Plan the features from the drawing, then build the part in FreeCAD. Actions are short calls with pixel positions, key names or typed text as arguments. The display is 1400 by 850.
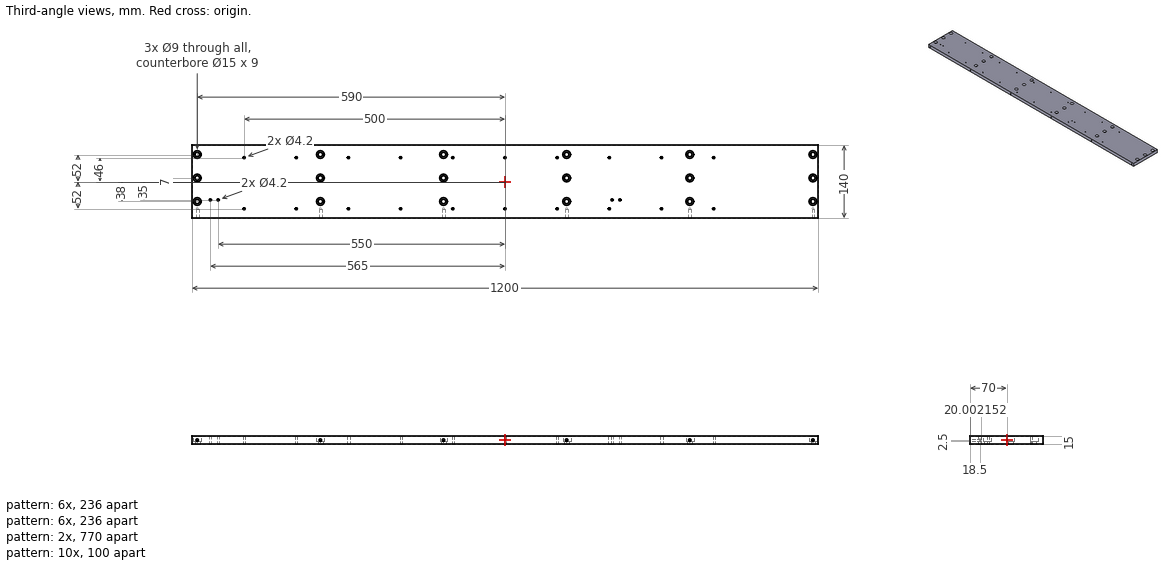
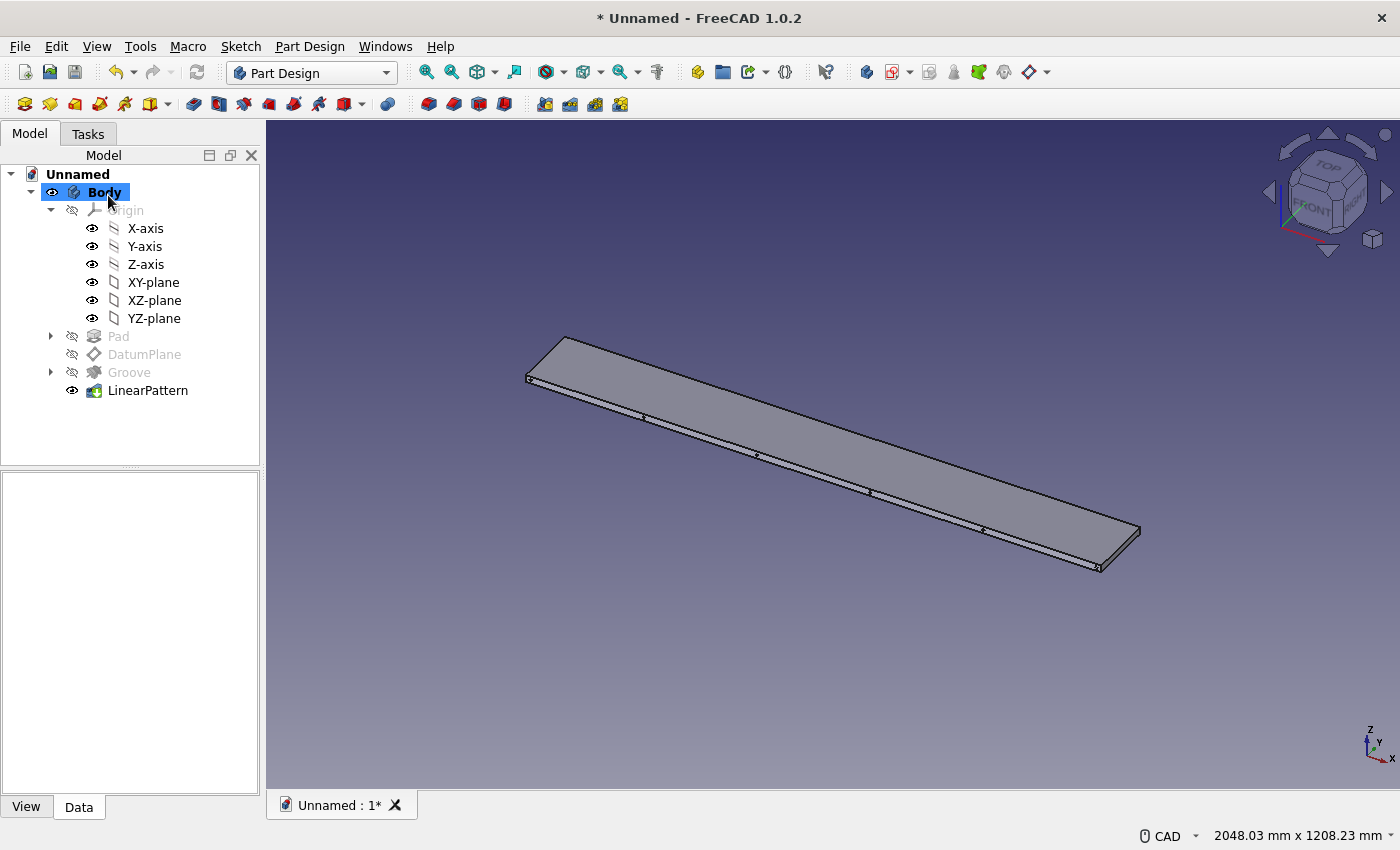
click(1080, 532)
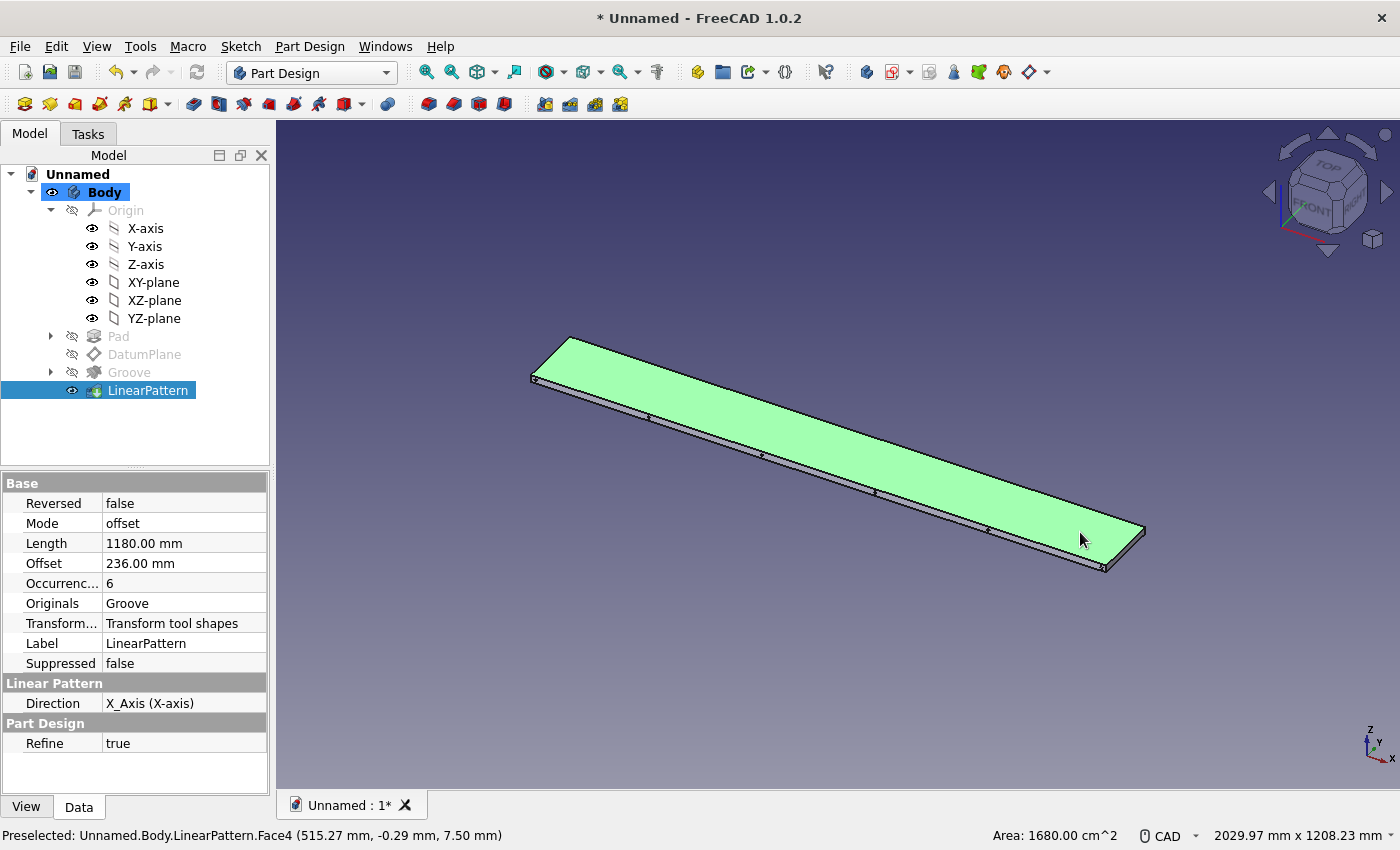
click(892, 72)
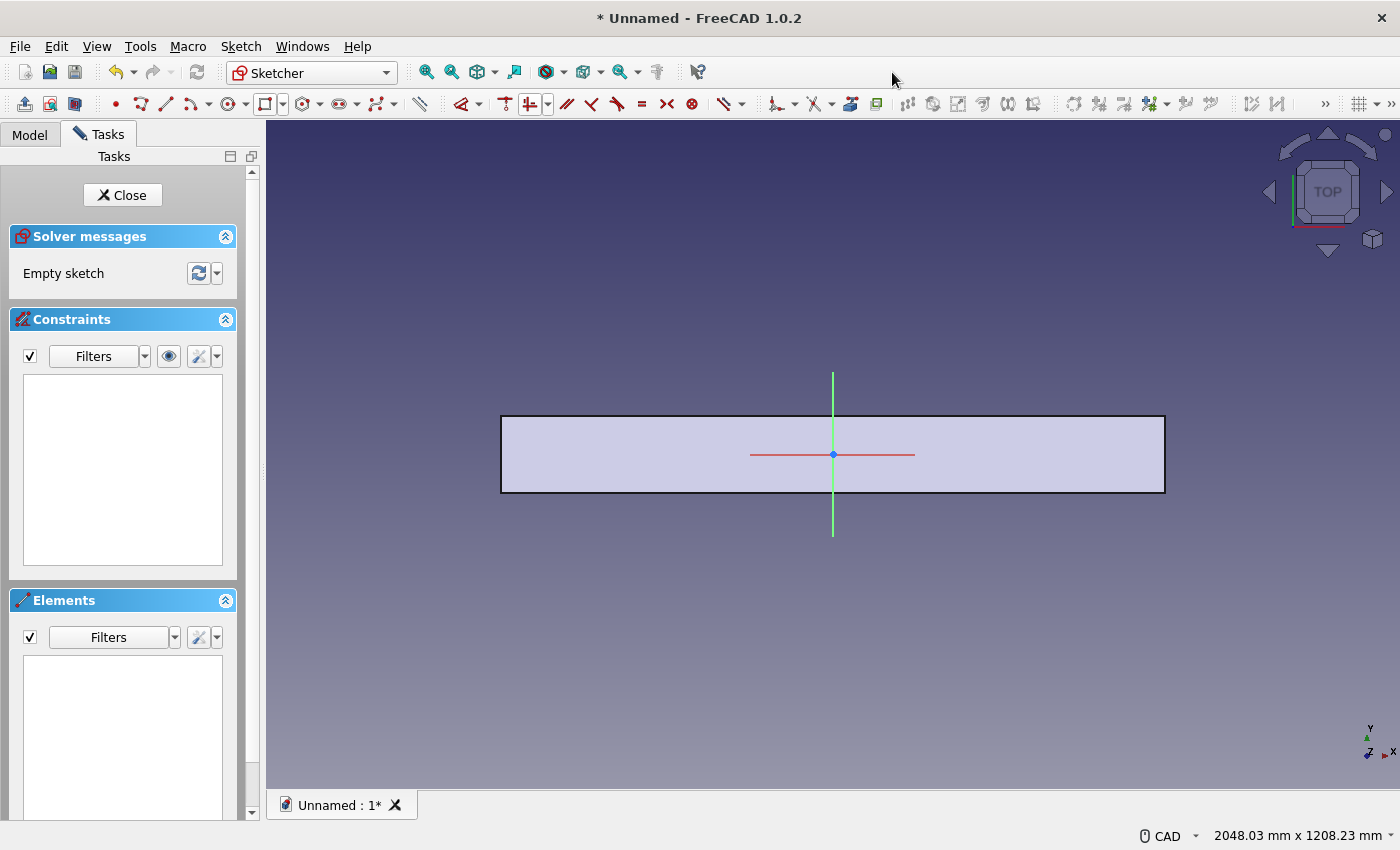
scroll(466, 450, up, 10)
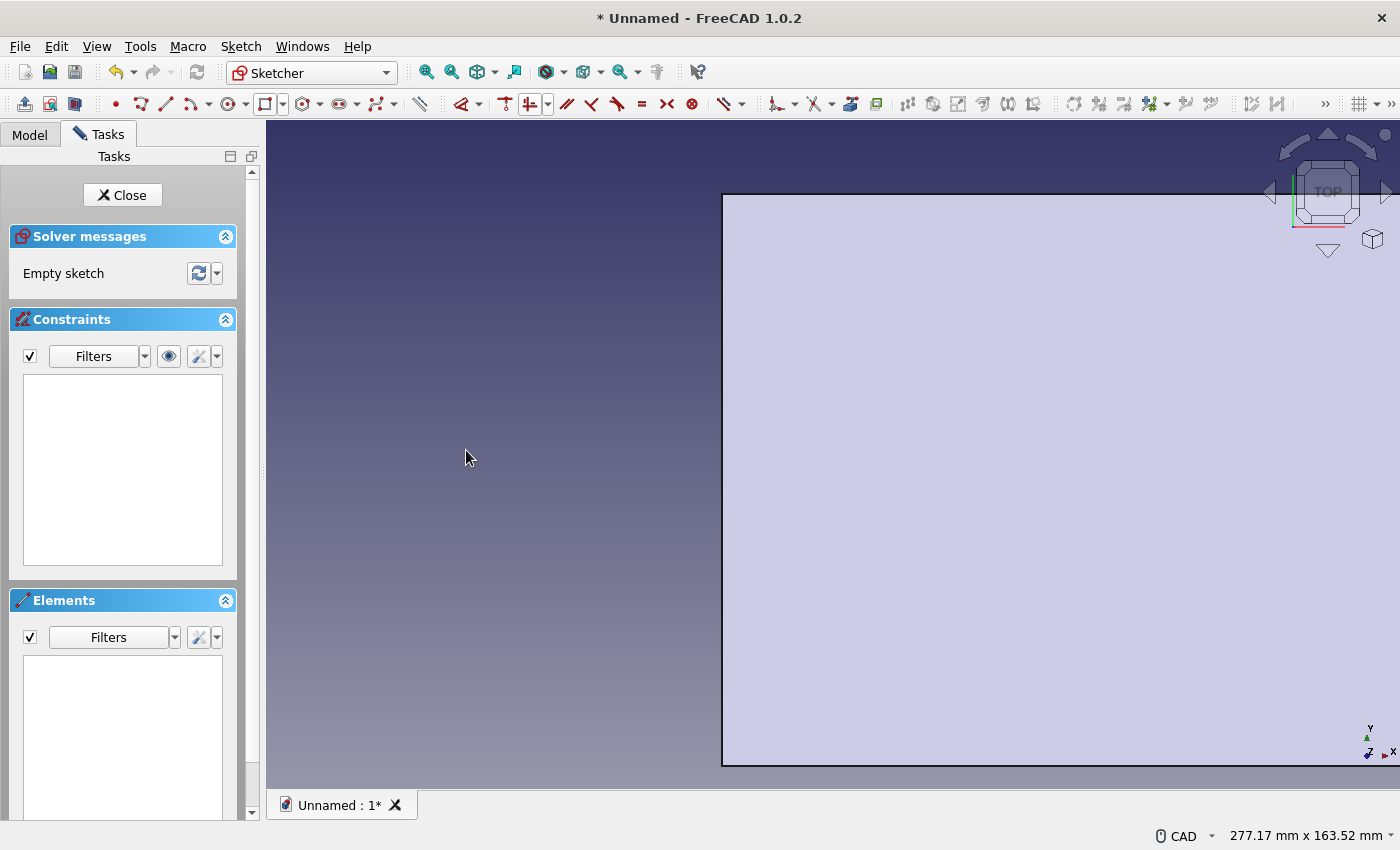
key(g)
key(c)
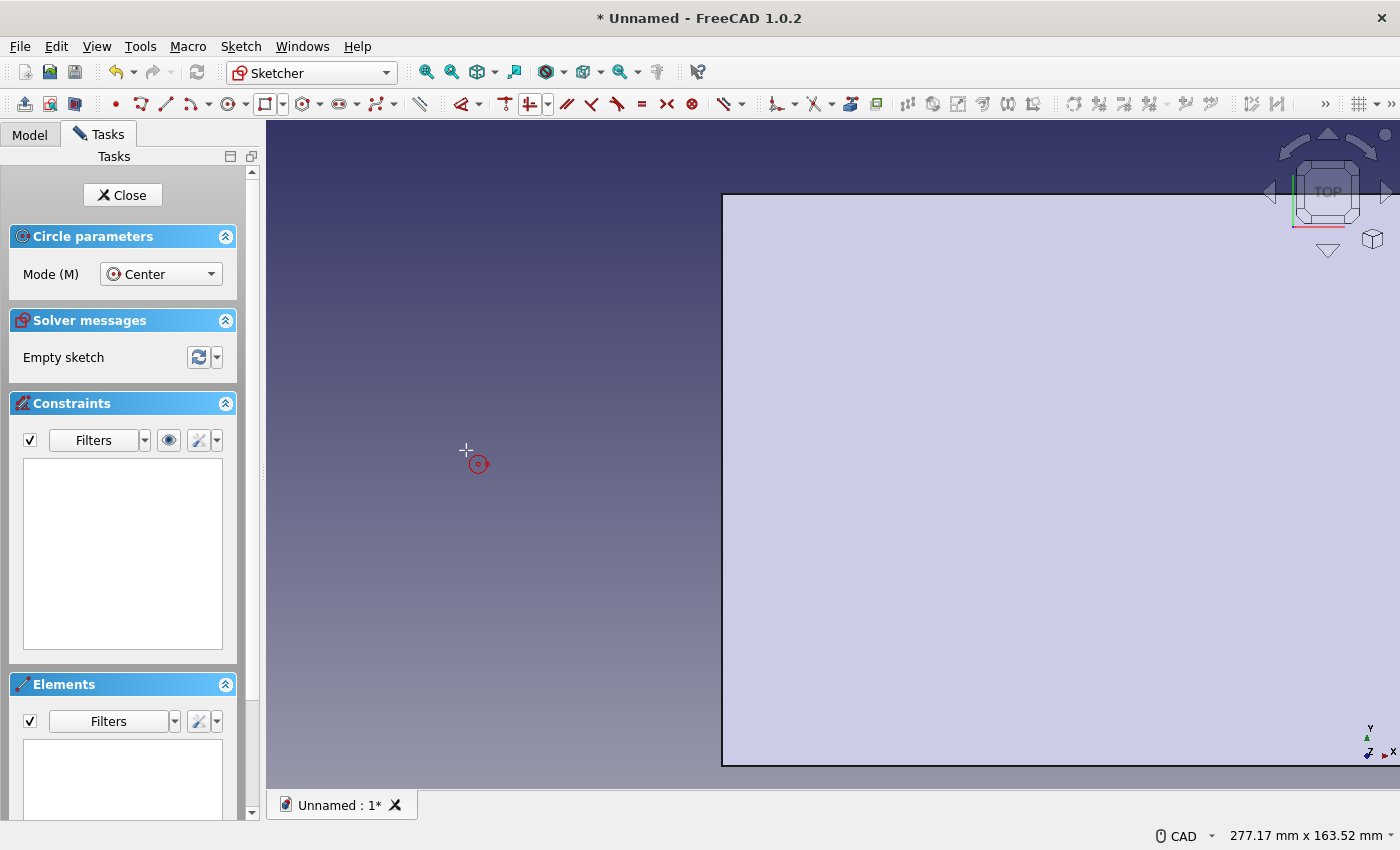
scroll(763, 267, up, 2)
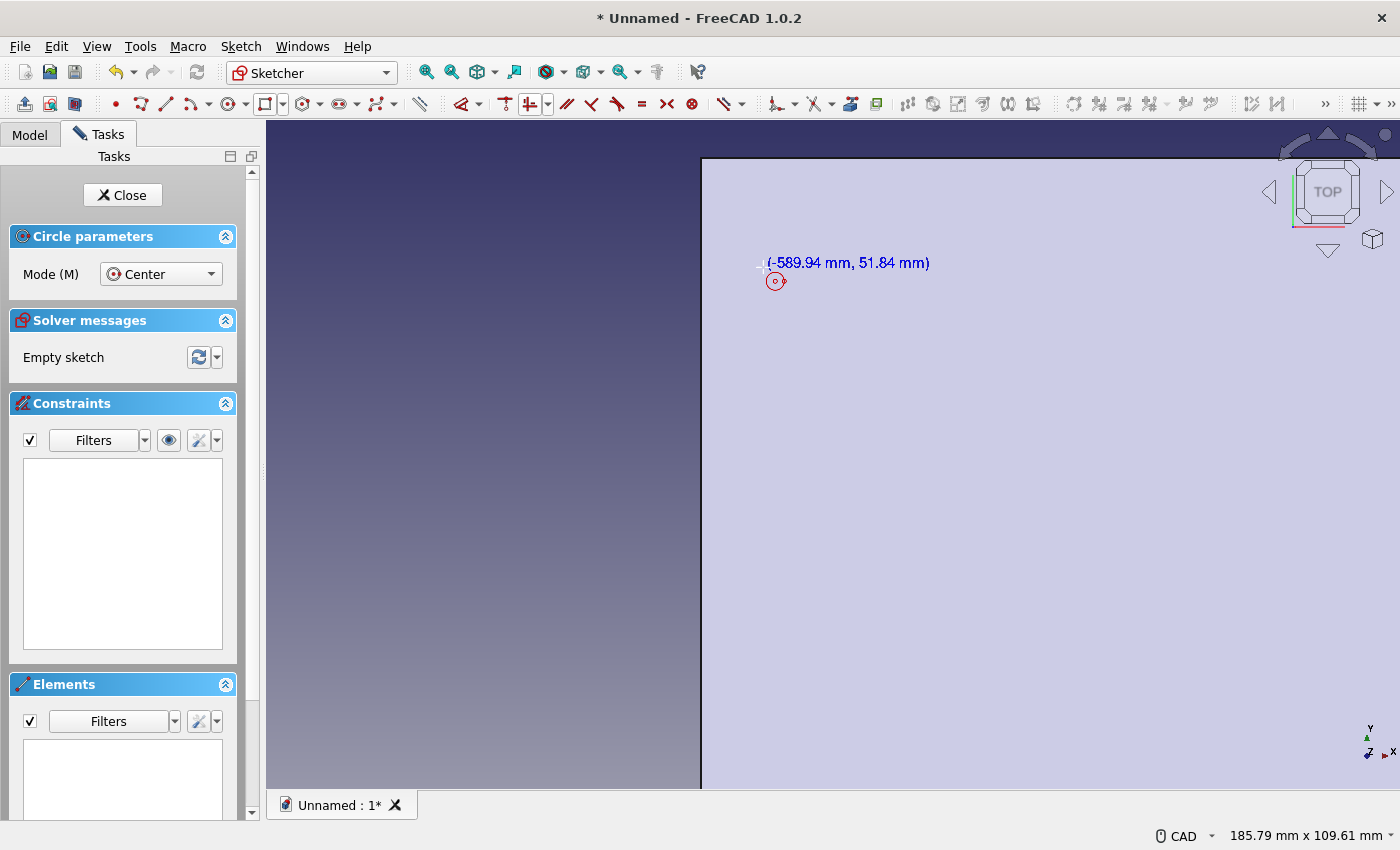
click(762, 267)
move(782, 248)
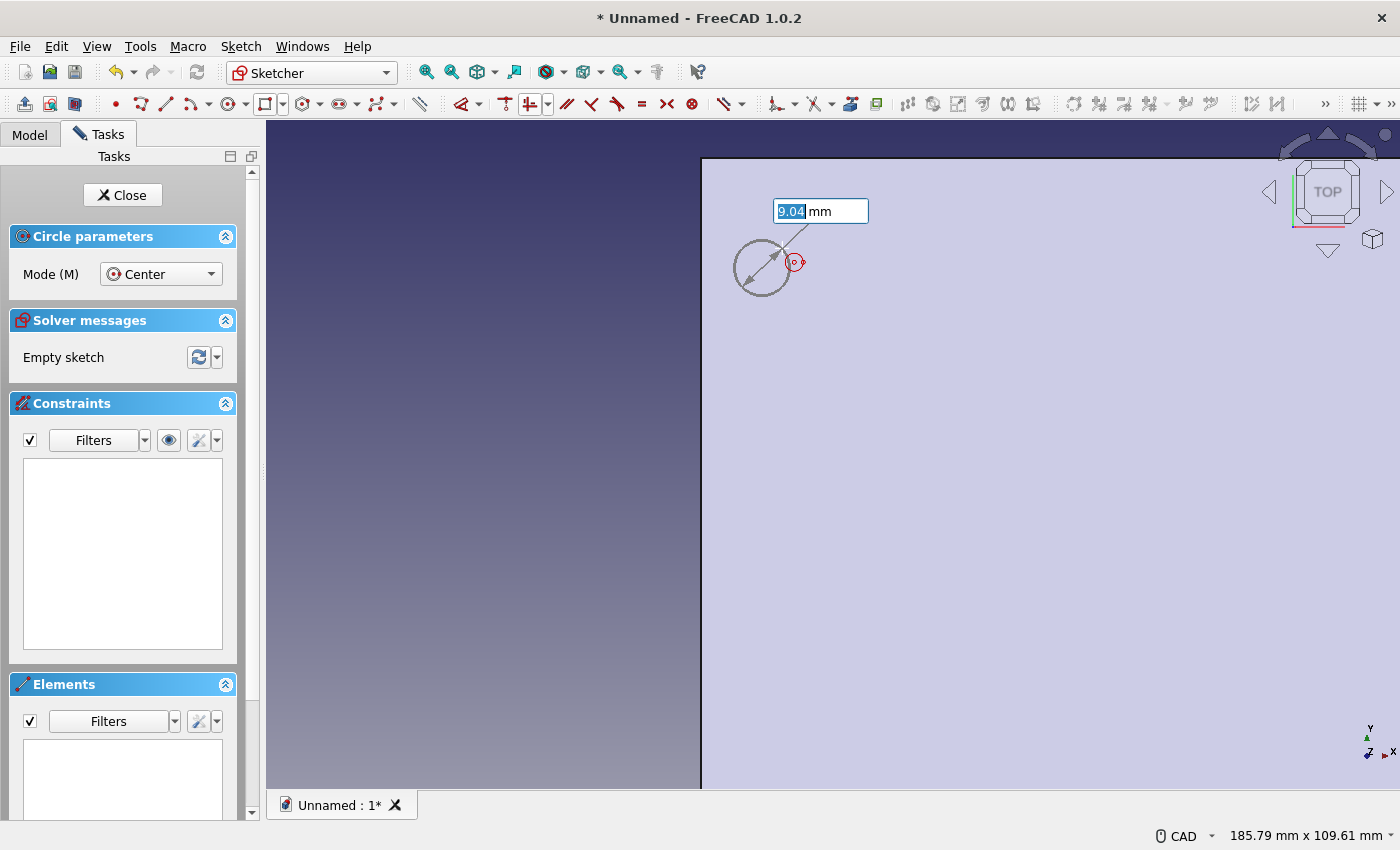
text(9)
key(Return)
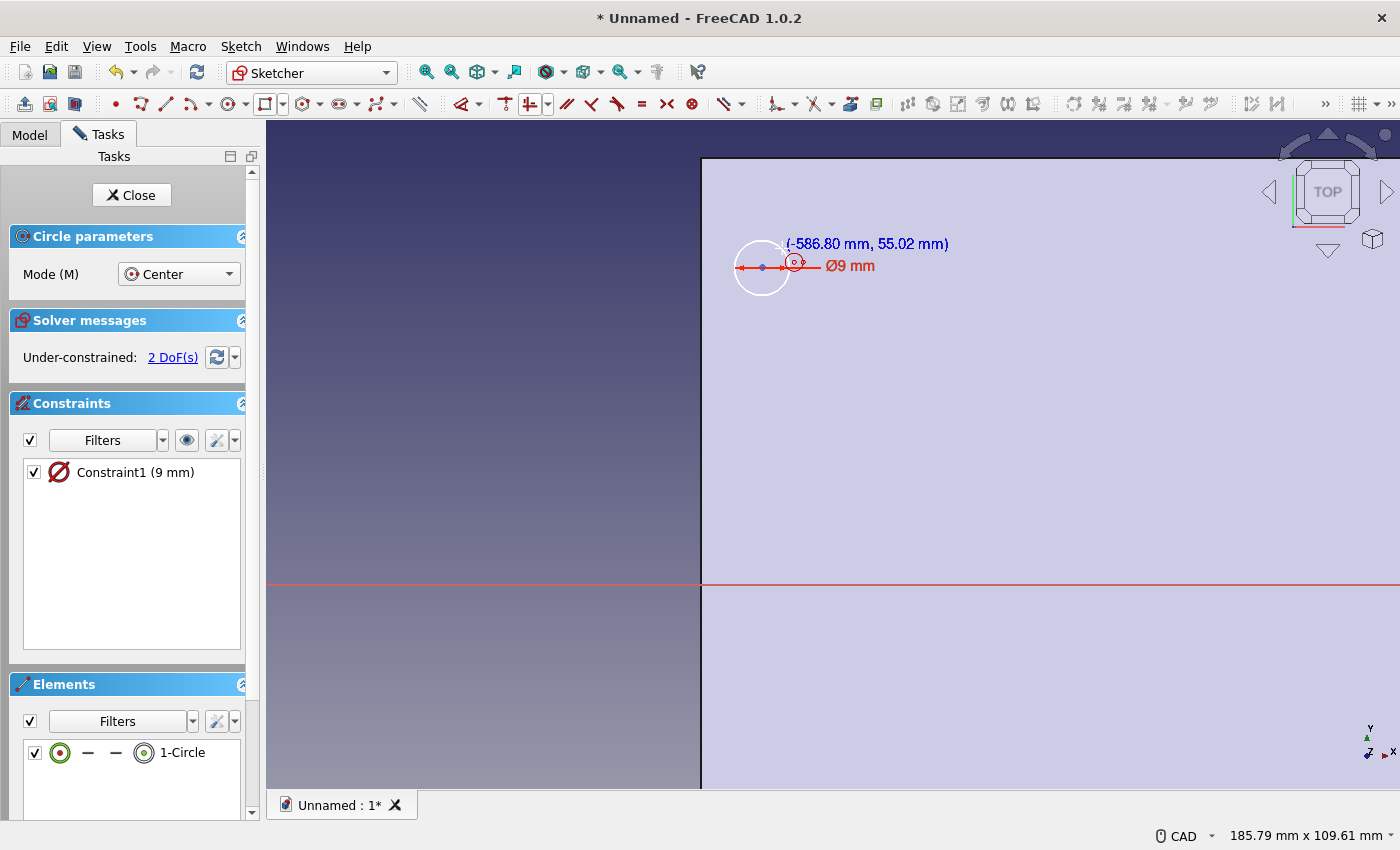
click(762, 542)
move(782, 523)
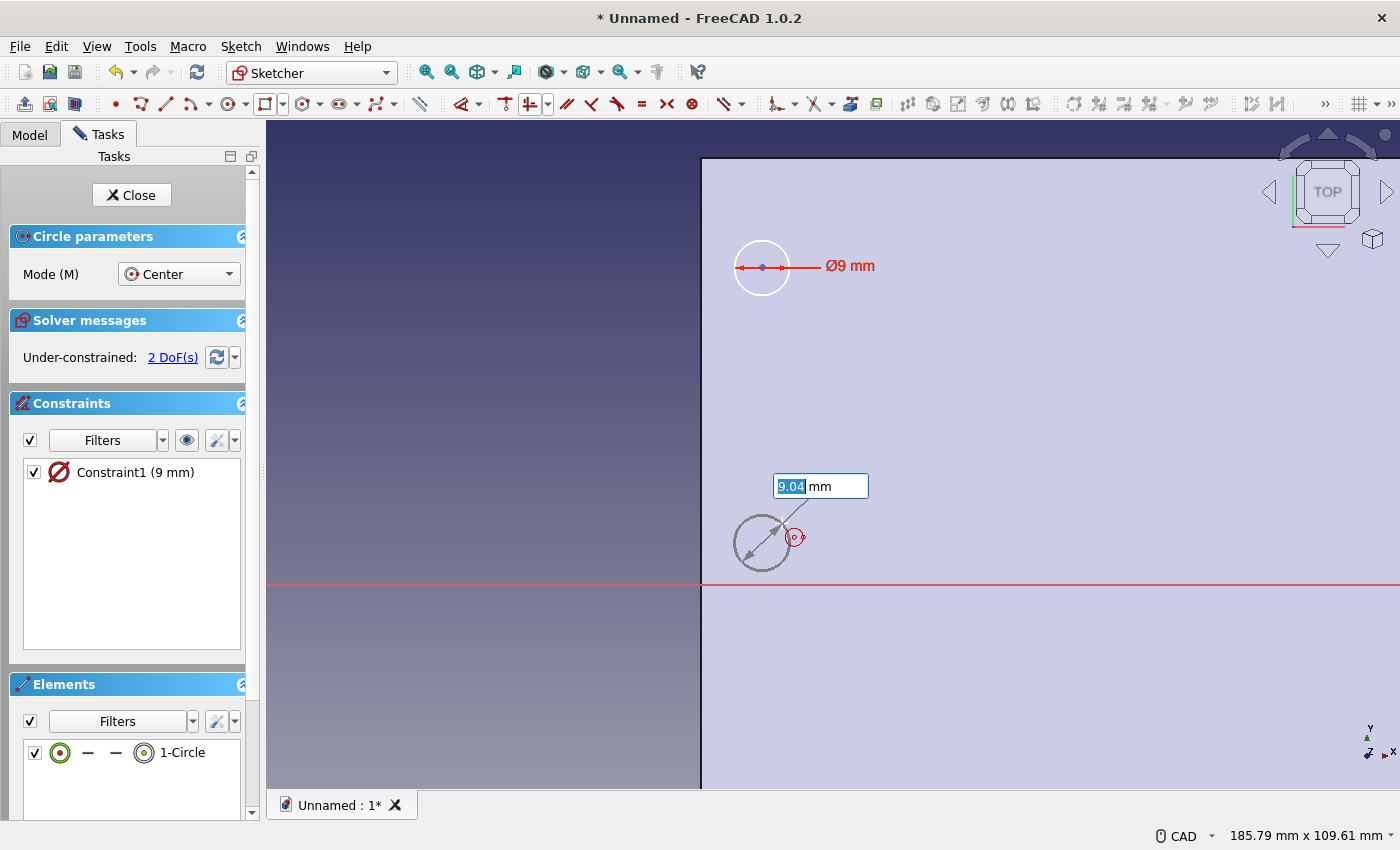
text(9)
key(Return)